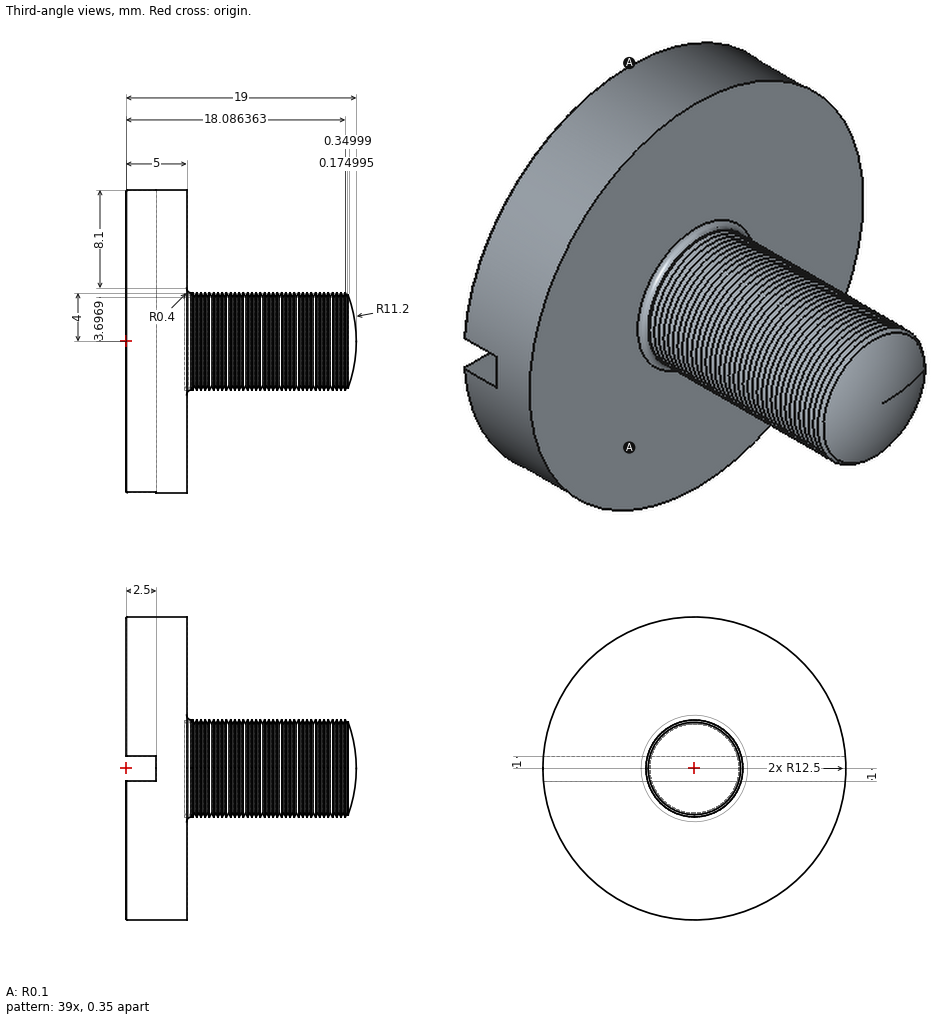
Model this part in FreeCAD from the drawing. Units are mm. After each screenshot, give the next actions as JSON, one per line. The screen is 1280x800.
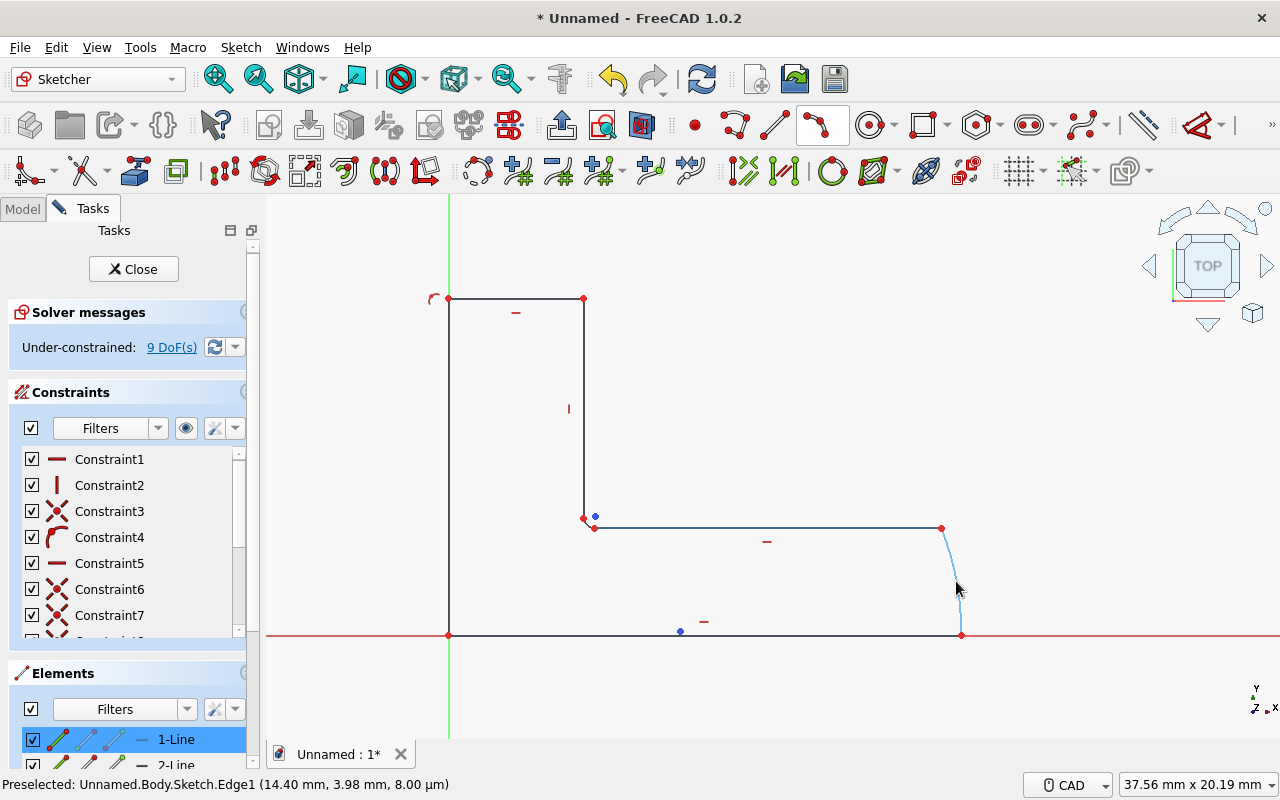
{"action": "scroll", "coordinate": [585, 523], "scroll_direction": "up", "scroll_amount": 6}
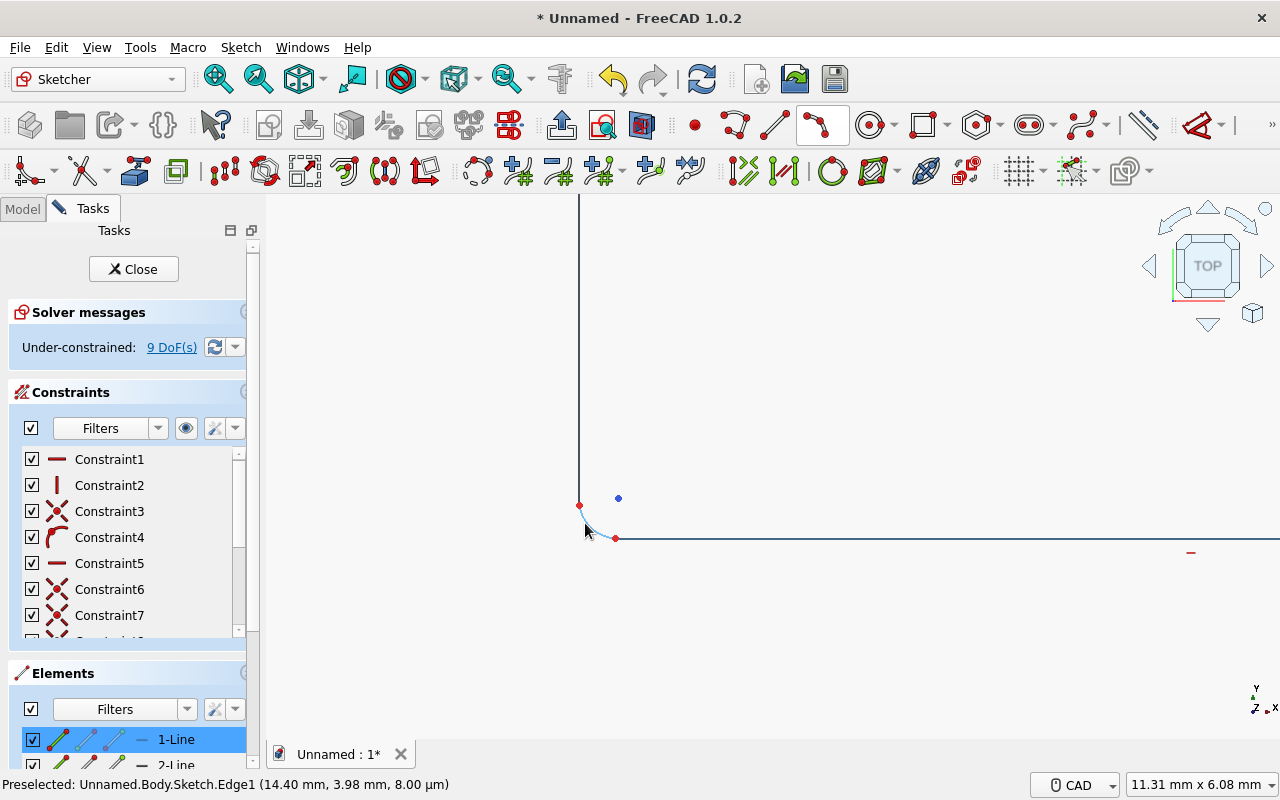
{"action": "left_click", "coordinate": [585, 520]}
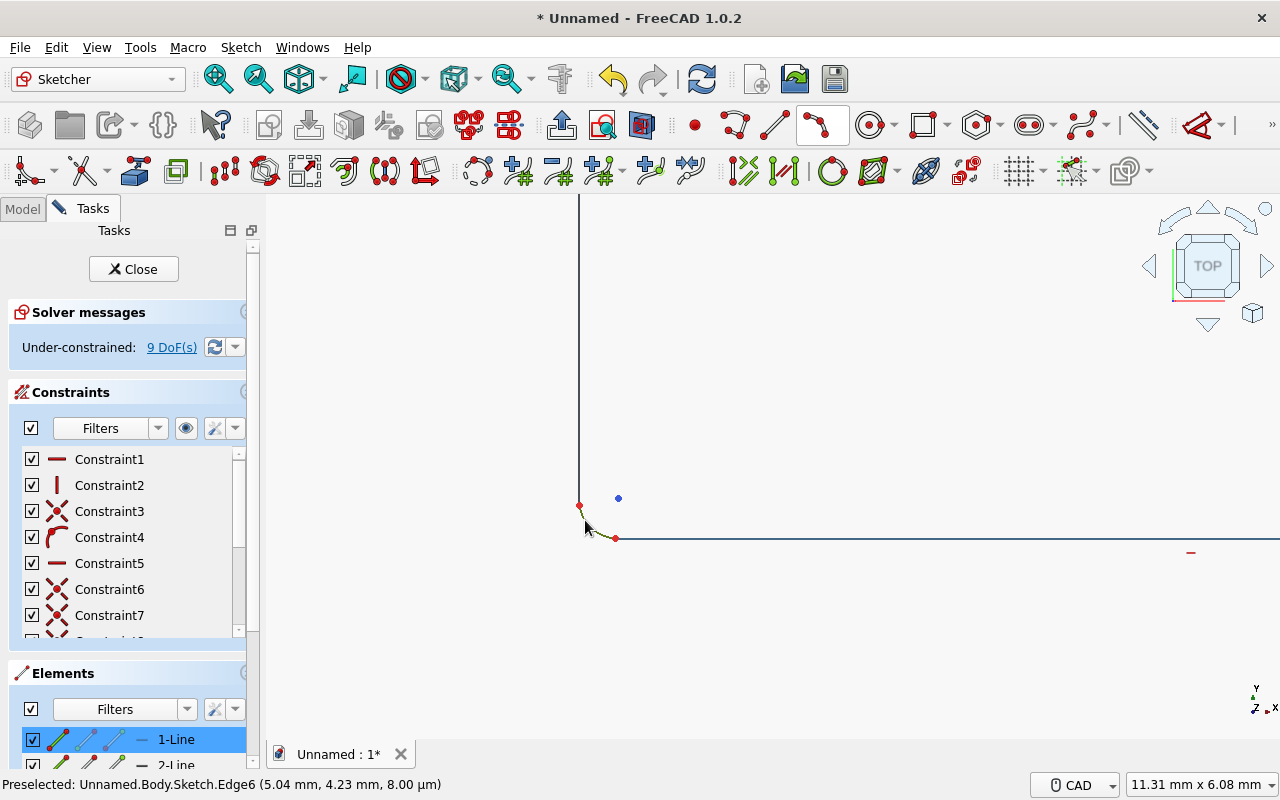
{"action": "key", "text": "t"}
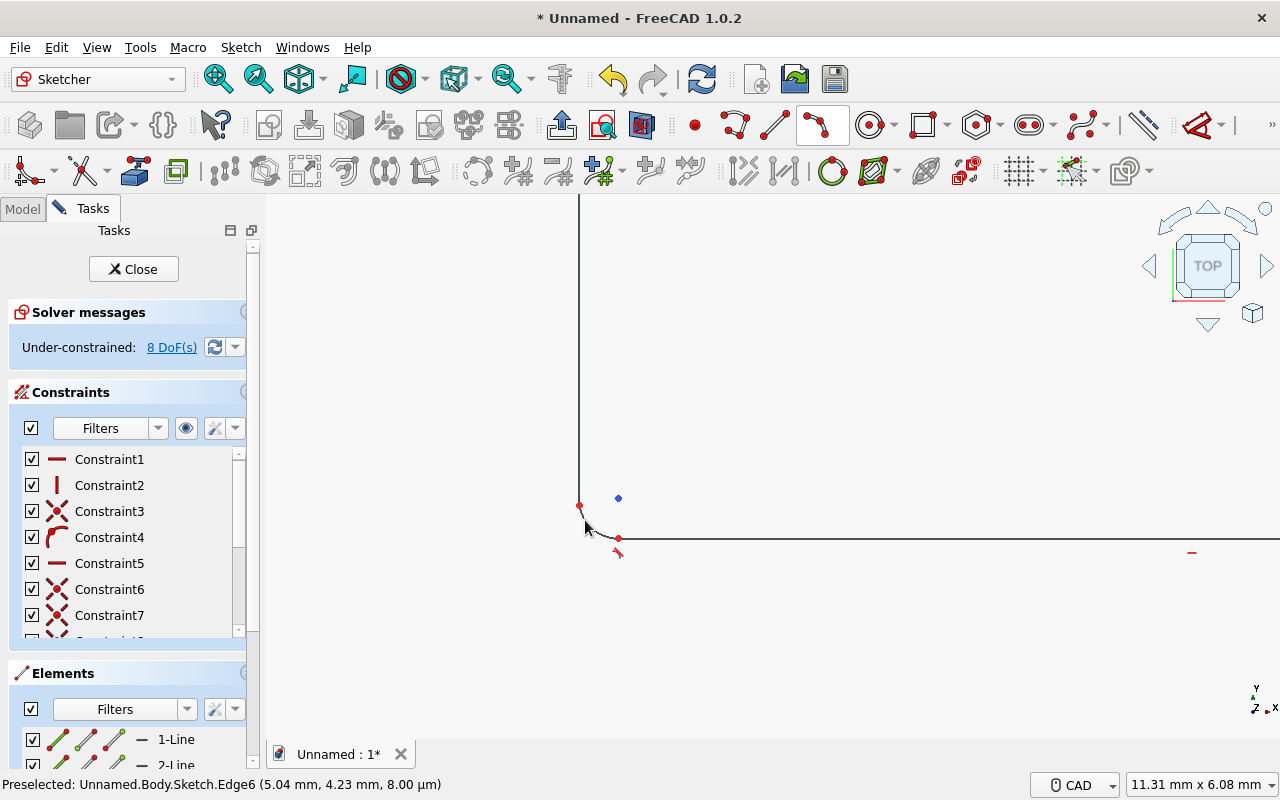
{"action": "left_click", "coordinate": [579, 287]}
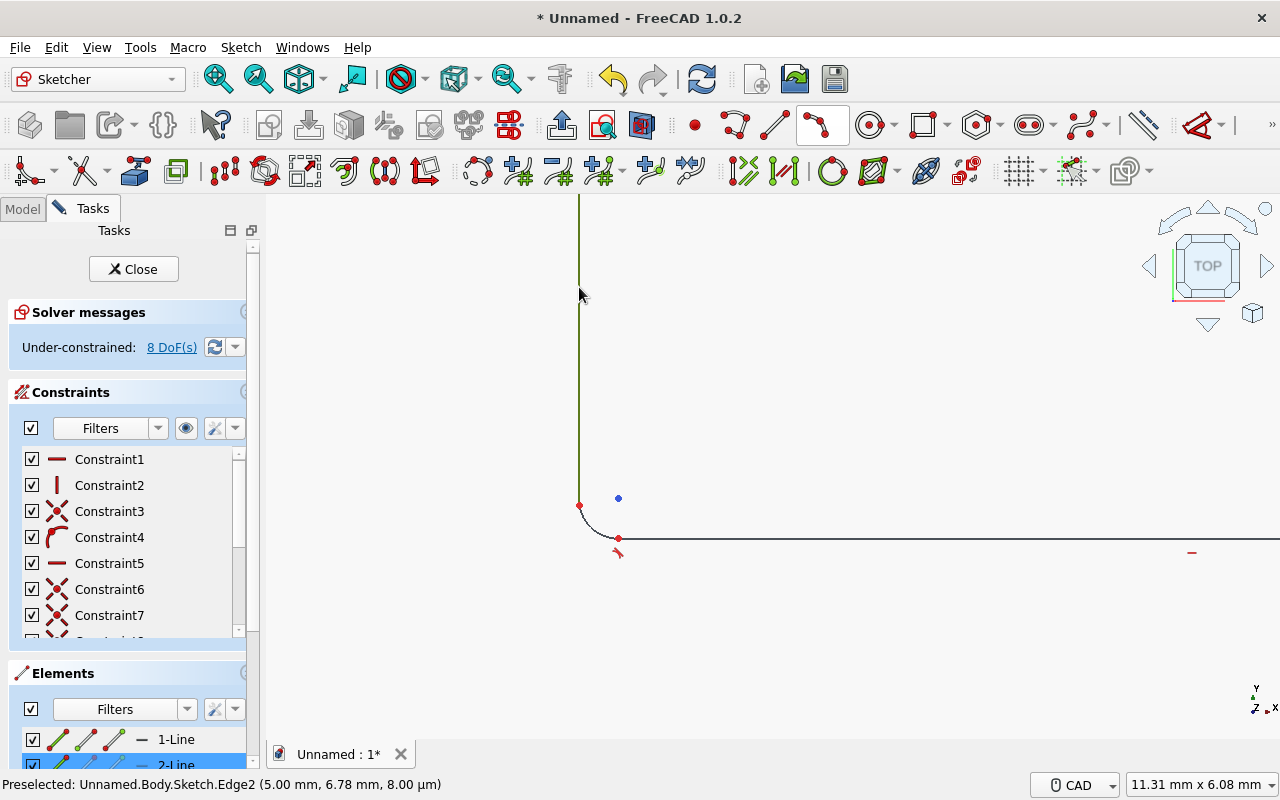
{"action": "left_click", "coordinate": [586, 521]}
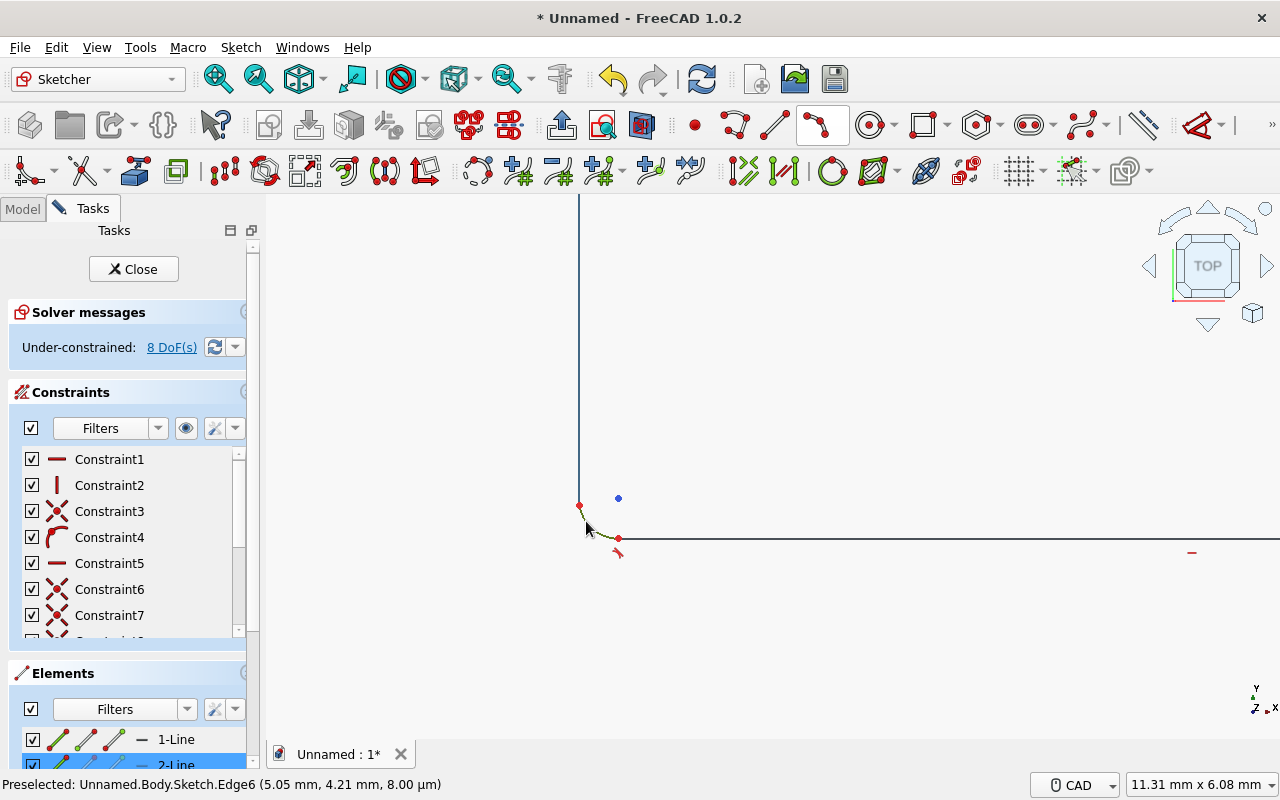
{"action": "key", "text": "t"}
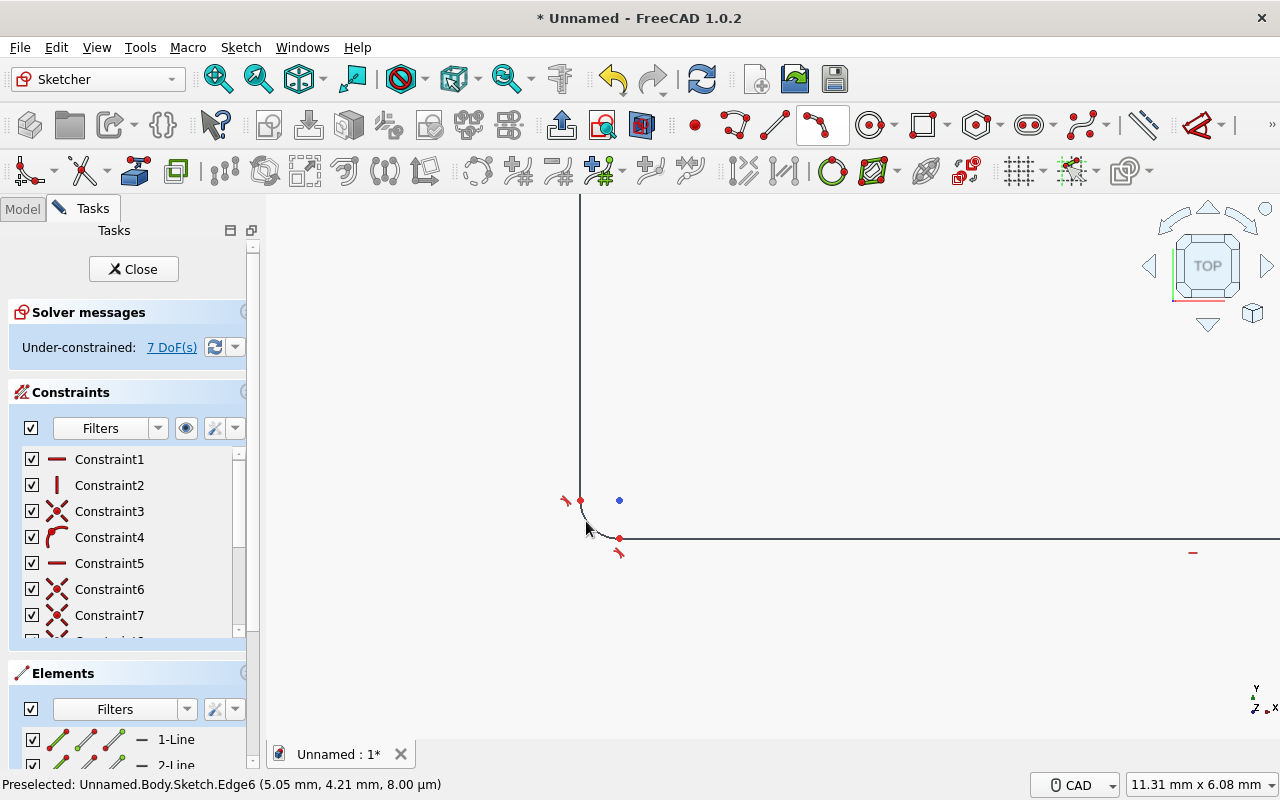
{"action": "scroll", "coordinate": [585, 523], "scroll_direction": "down", "scroll_amount": 6}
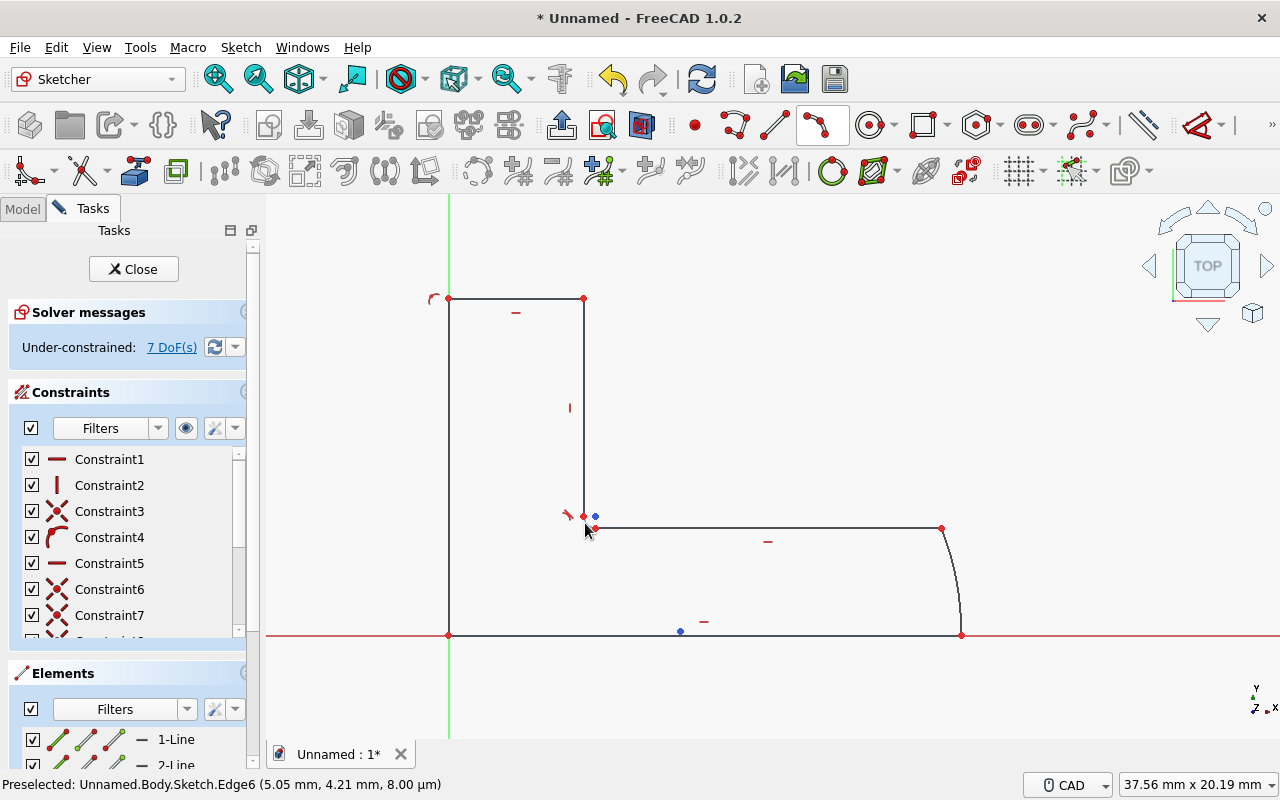
{"action": "left_click", "coordinate": [681, 632]}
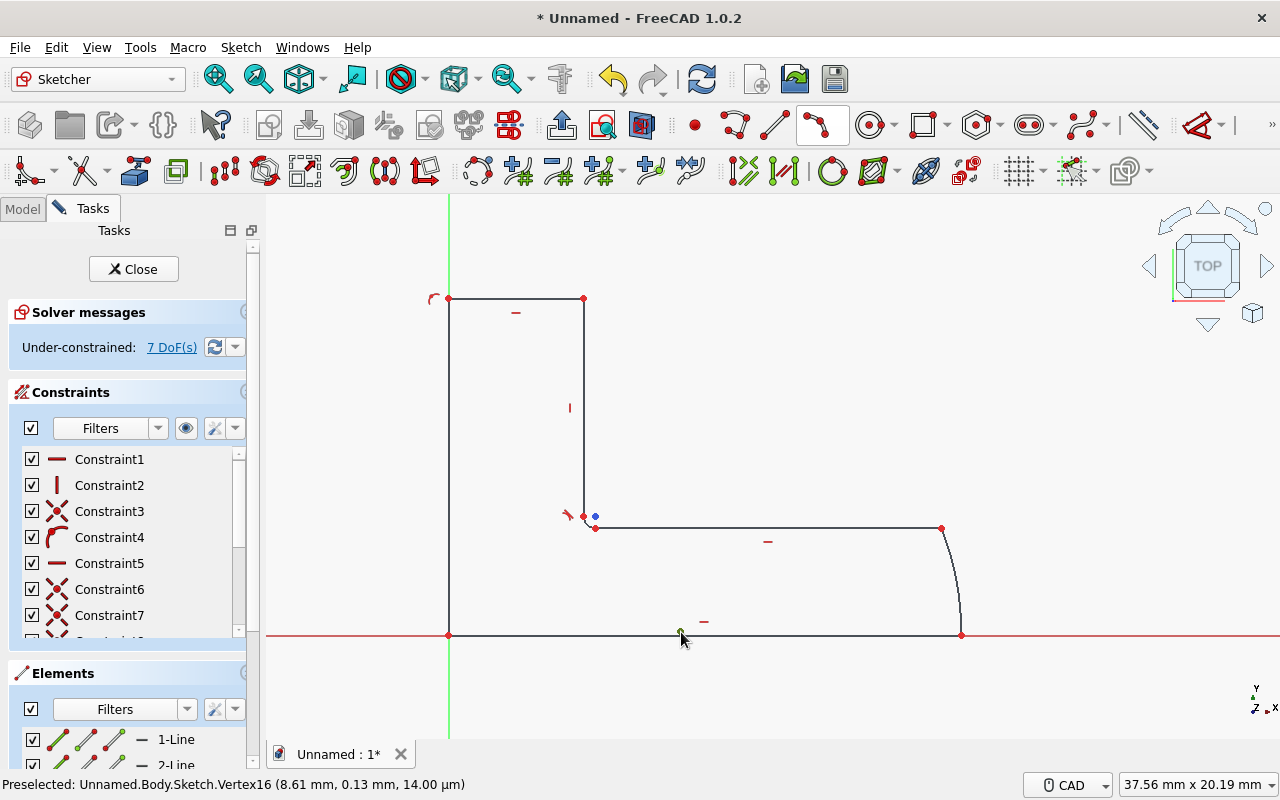
{"action": "left_click", "coordinate": [353, 636]}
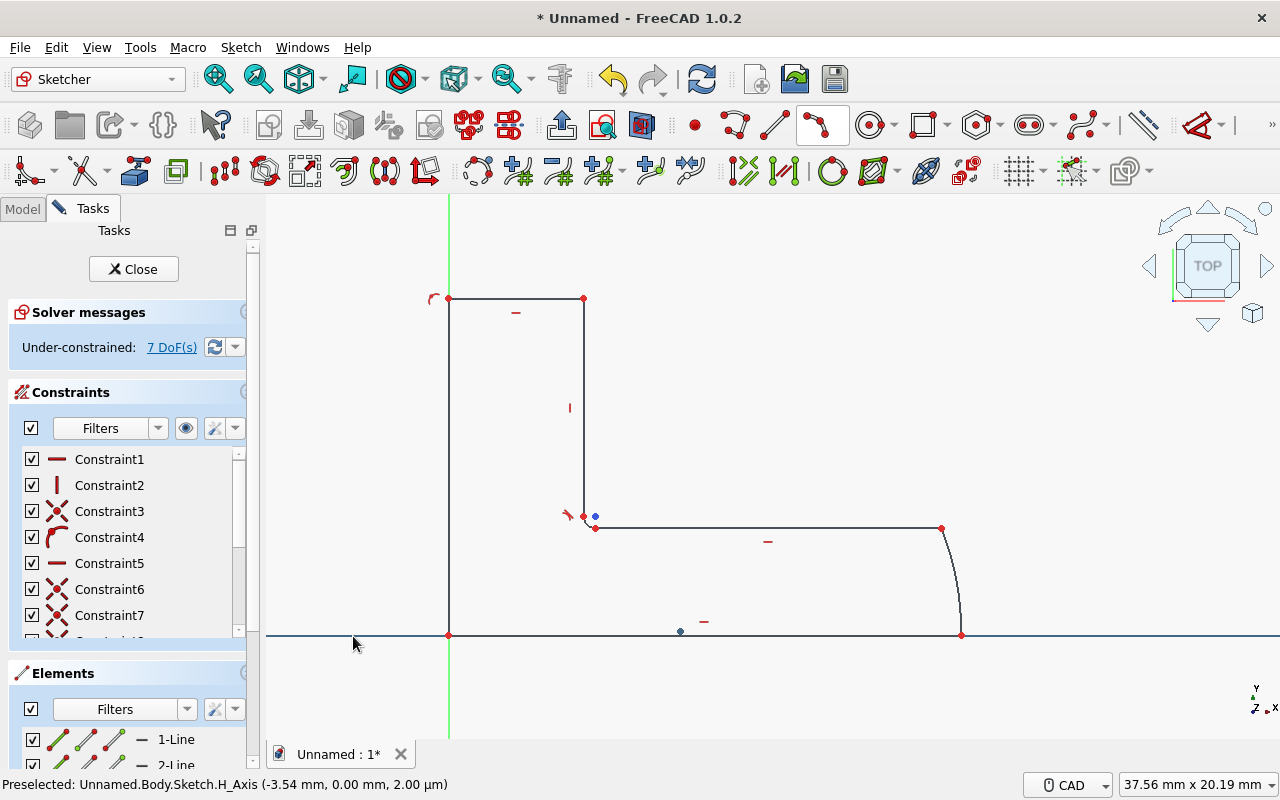
{"action": "key", "text": "c"}